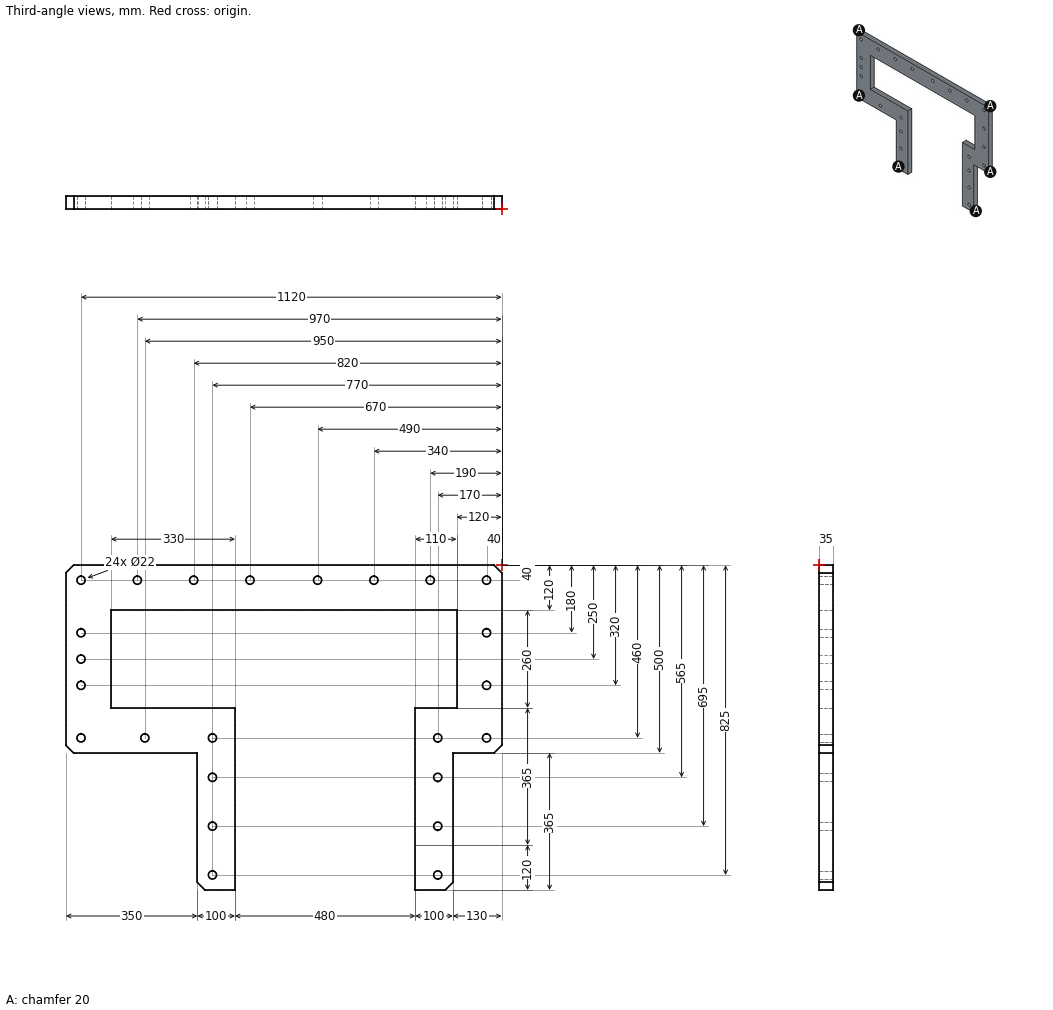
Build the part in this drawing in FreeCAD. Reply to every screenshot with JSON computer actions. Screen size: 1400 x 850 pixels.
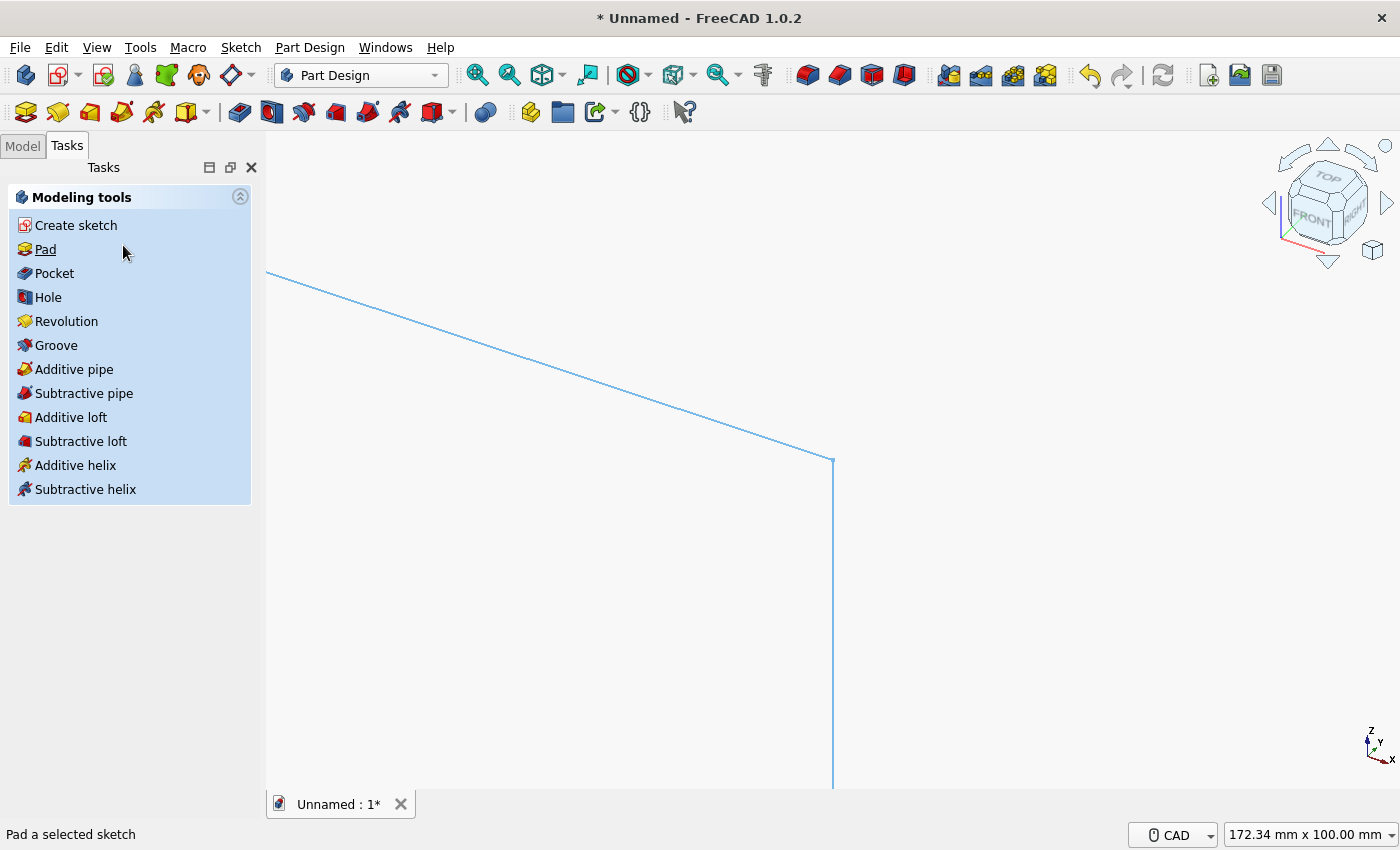
{"action": "left_click", "coordinate": [26, 112]}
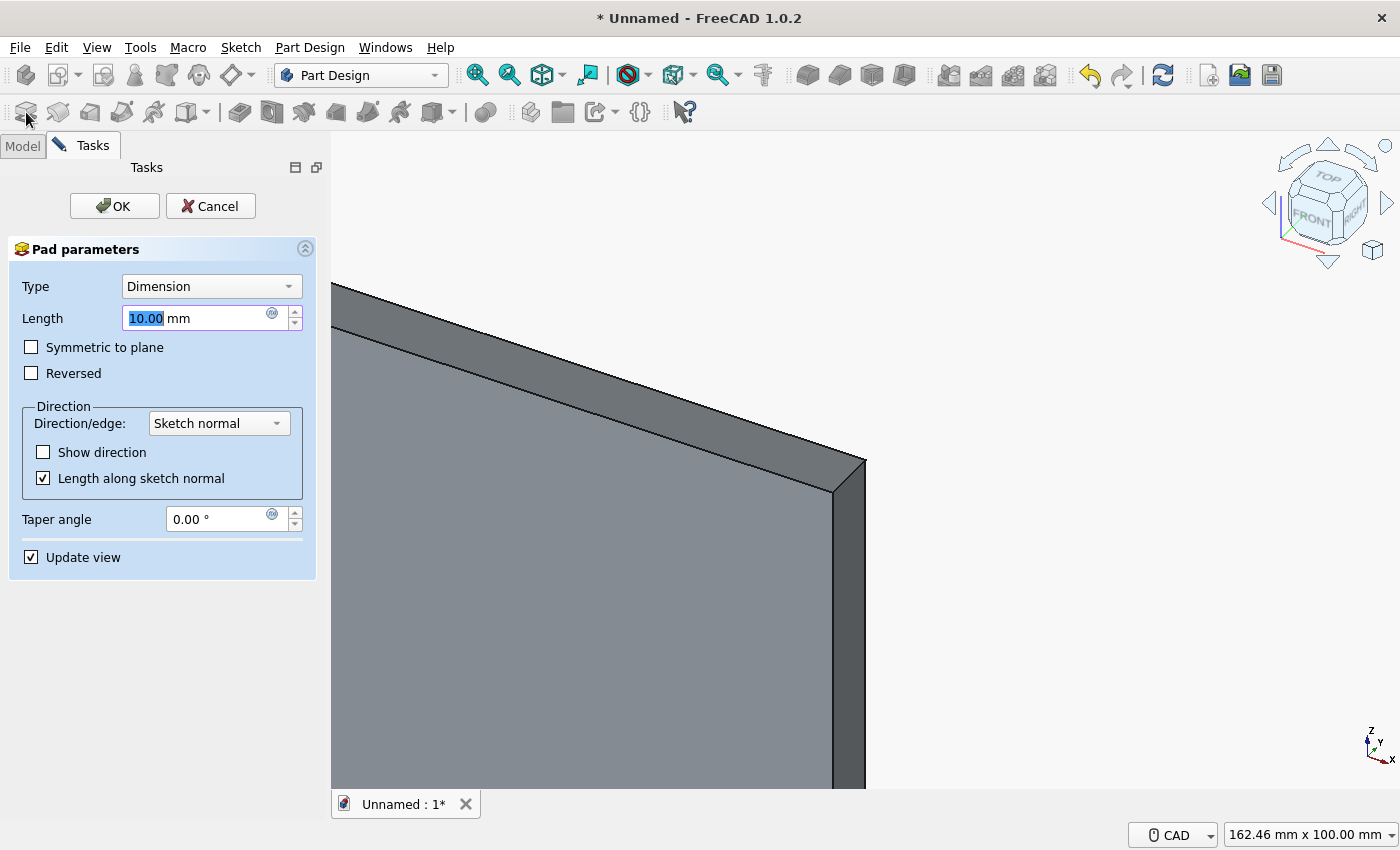
{"action": "type", "text": "35"}
{"action": "key", "text": "Tab"}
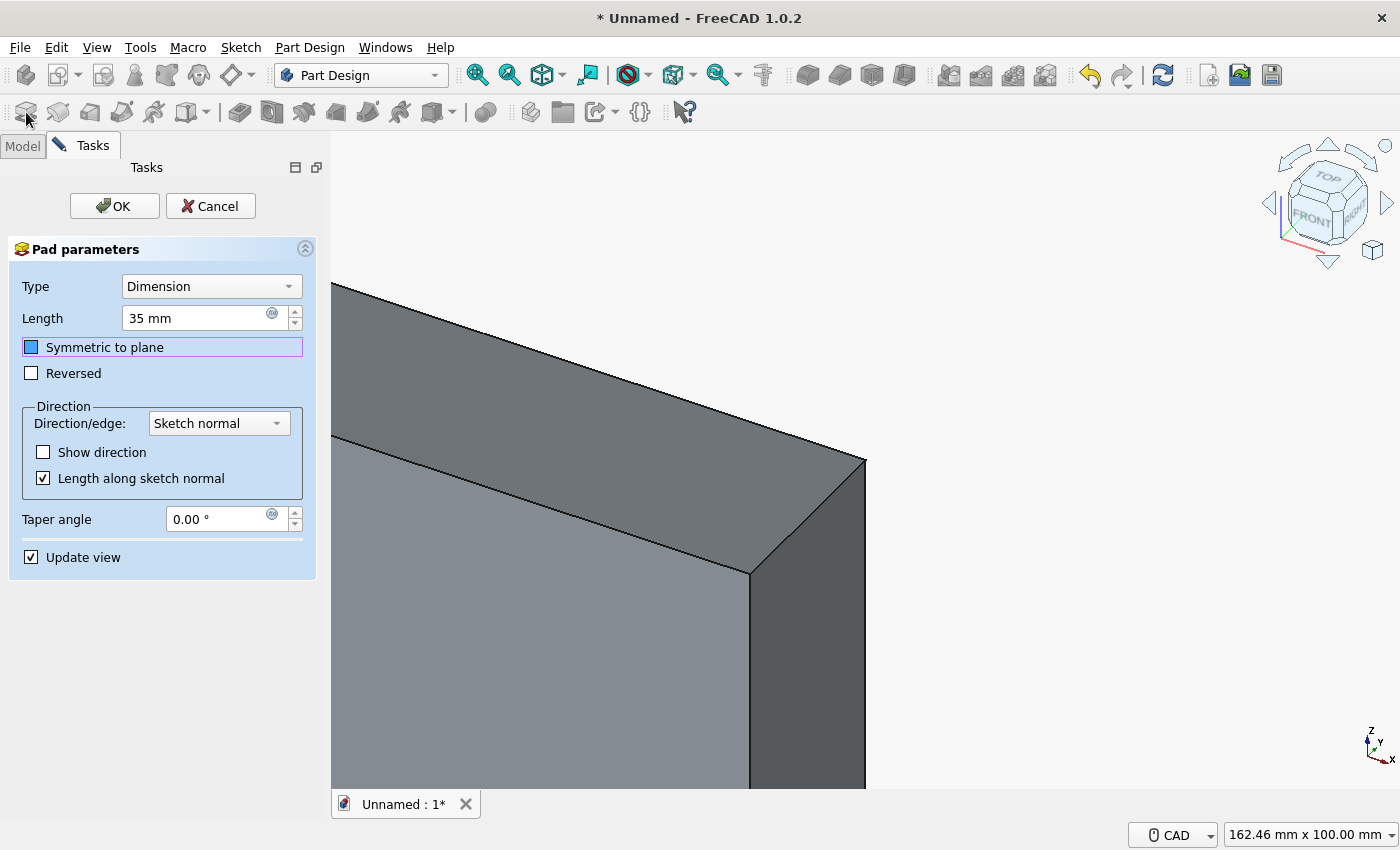
{"action": "left_click", "coordinate": [30, 373]}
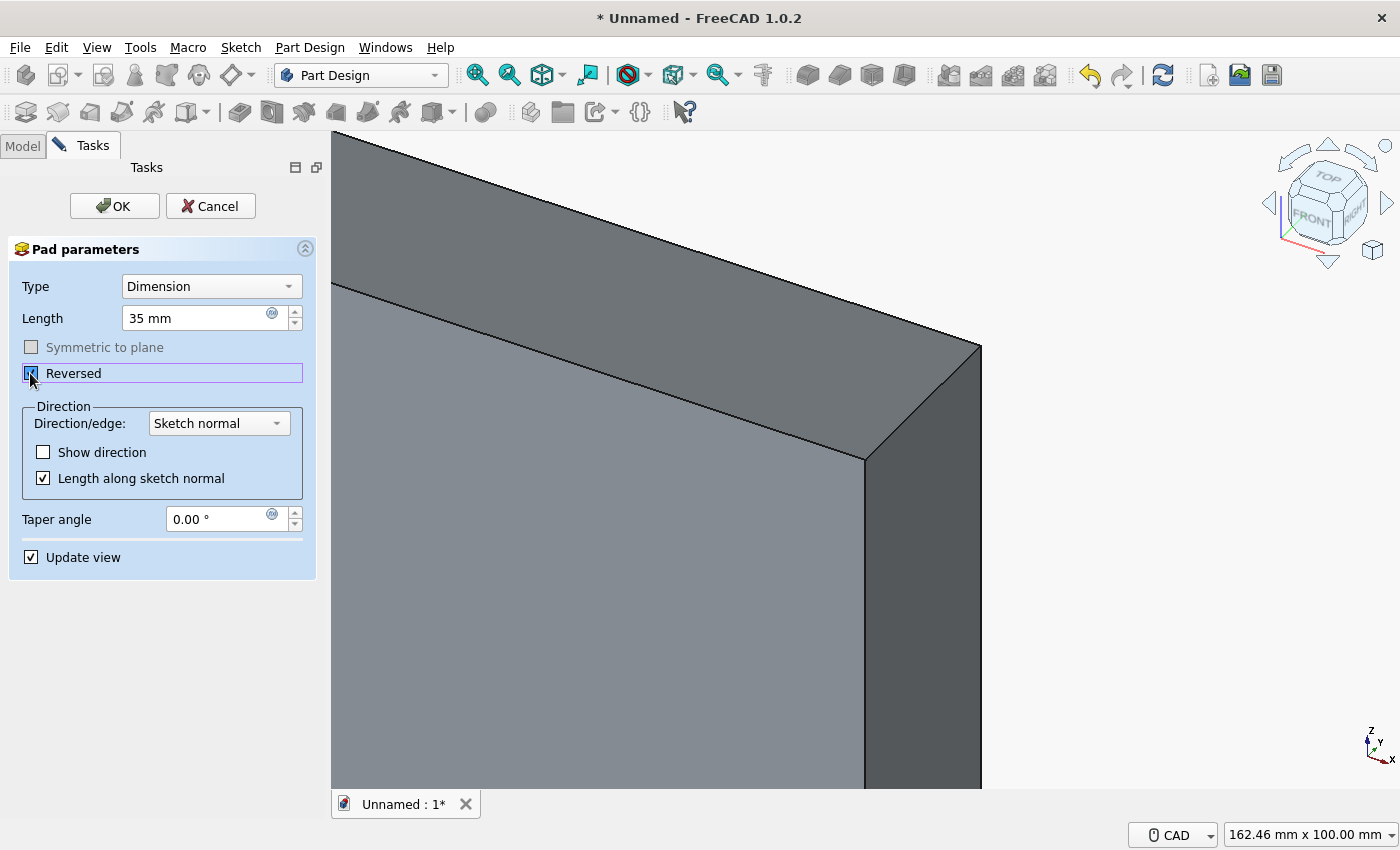
{"action": "left_click", "coordinate": [115, 206]}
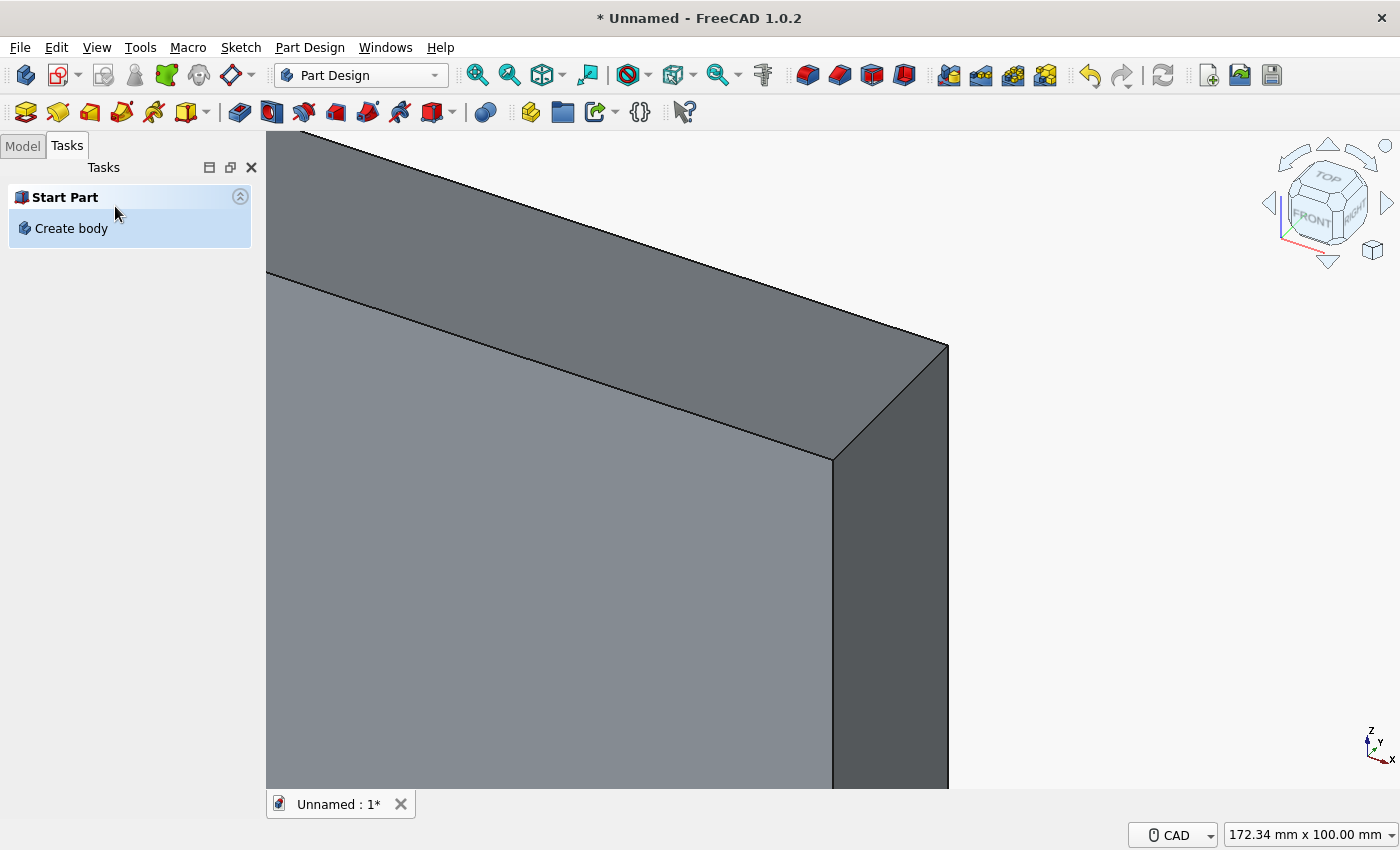
{"action": "key", "text": "v f"}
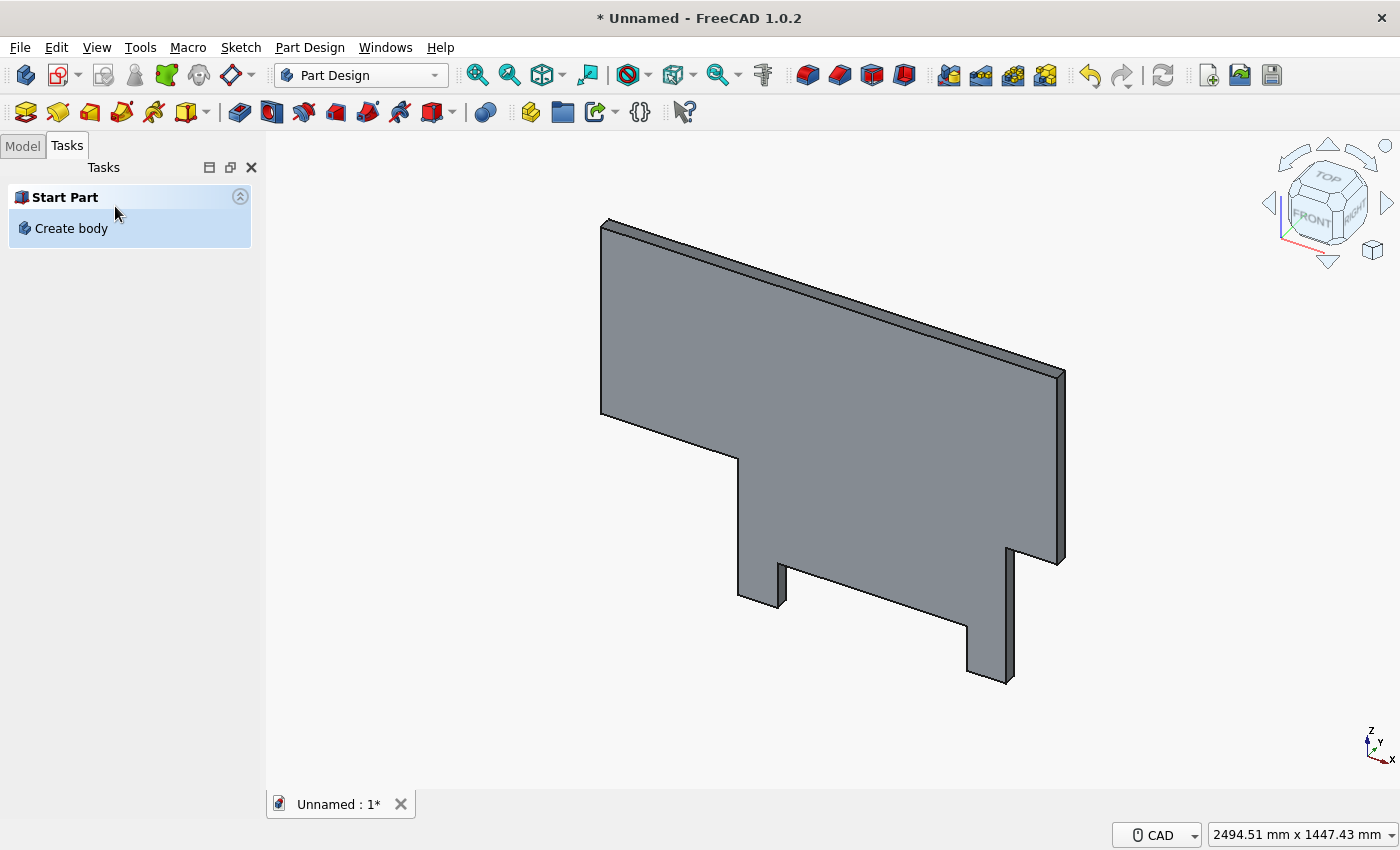
{"action": "key", "text": "4"}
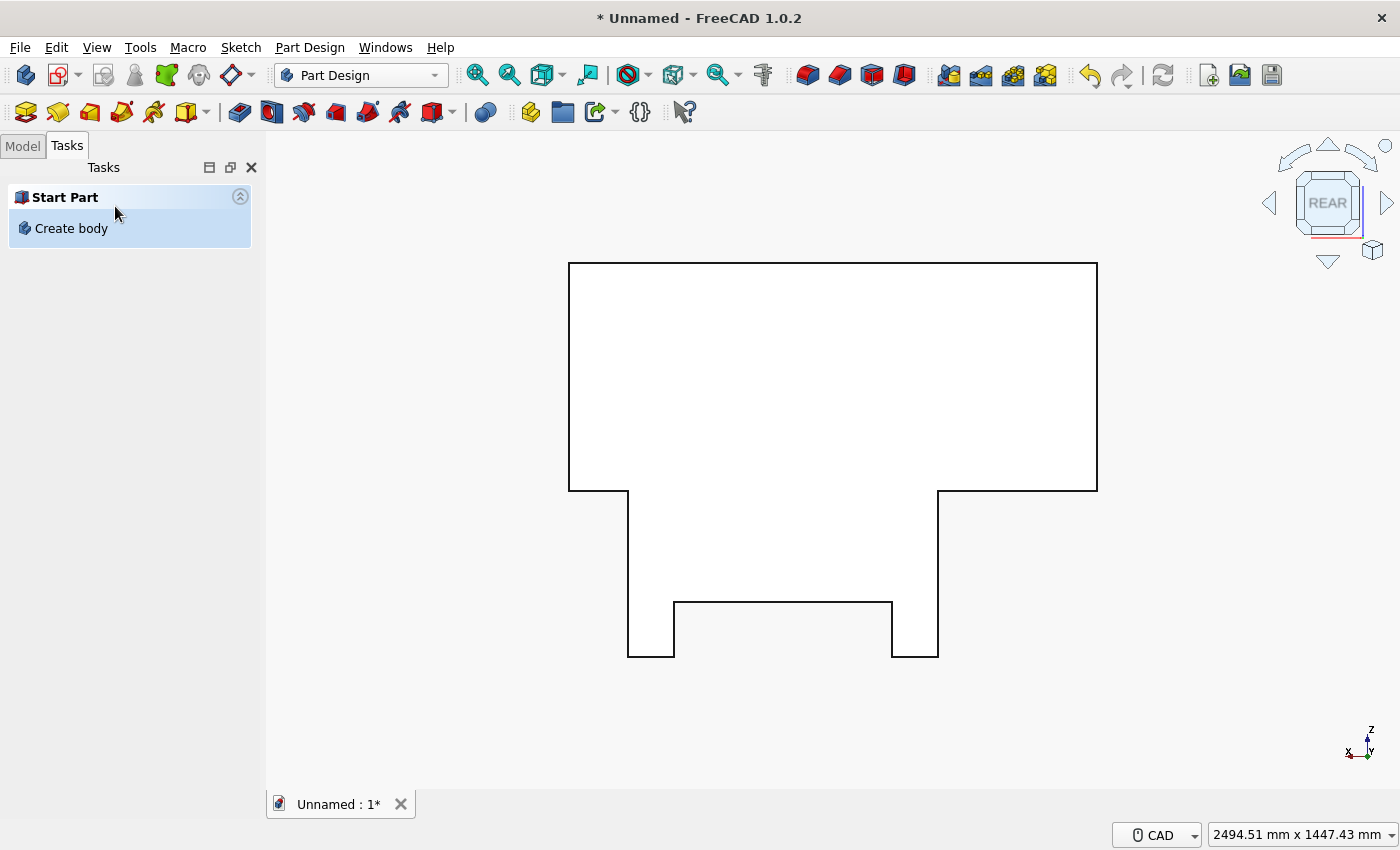
{"action": "left_click", "coordinate": [758, 403]}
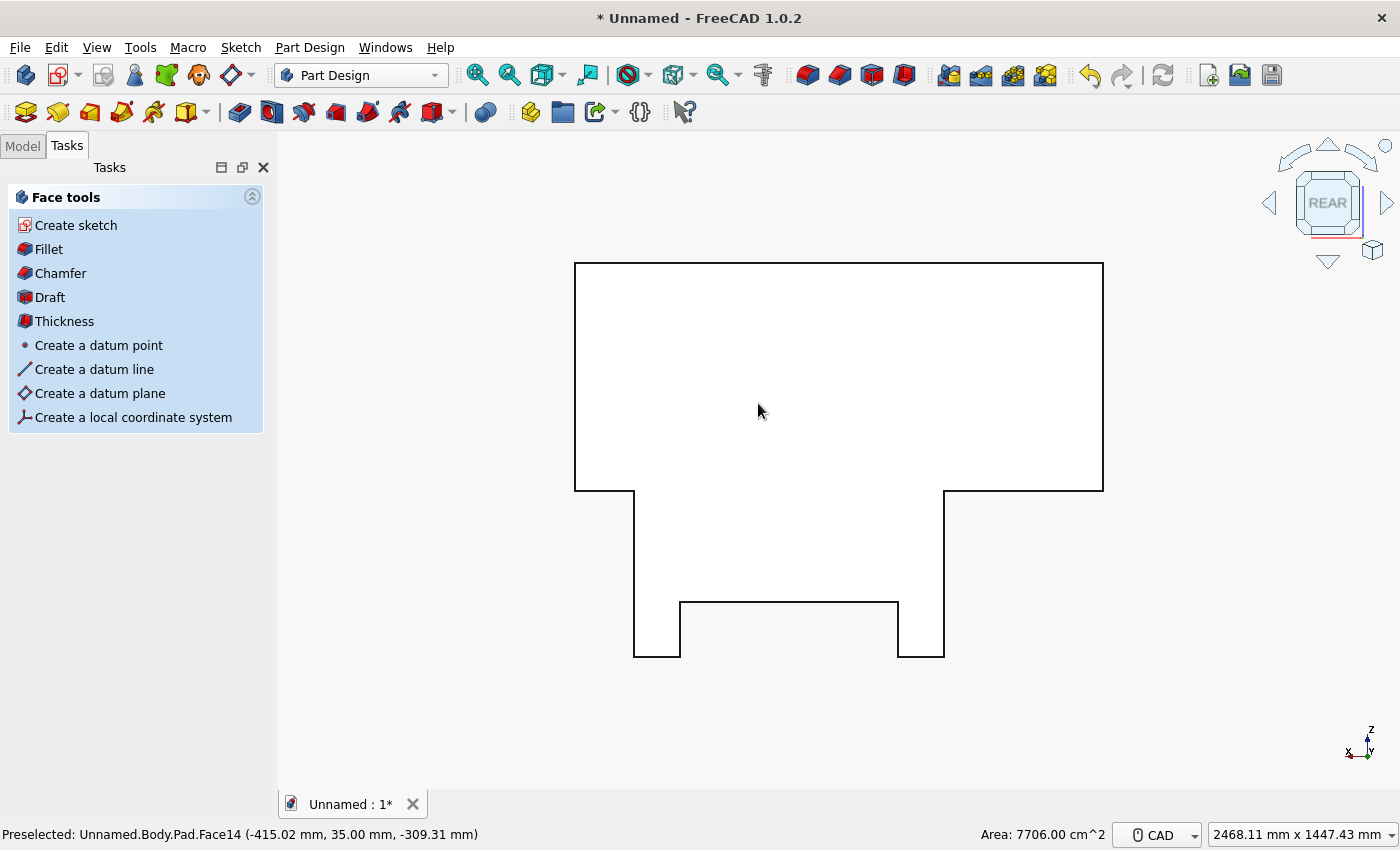
{"action": "left_click", "coordinate": [58, 76]}